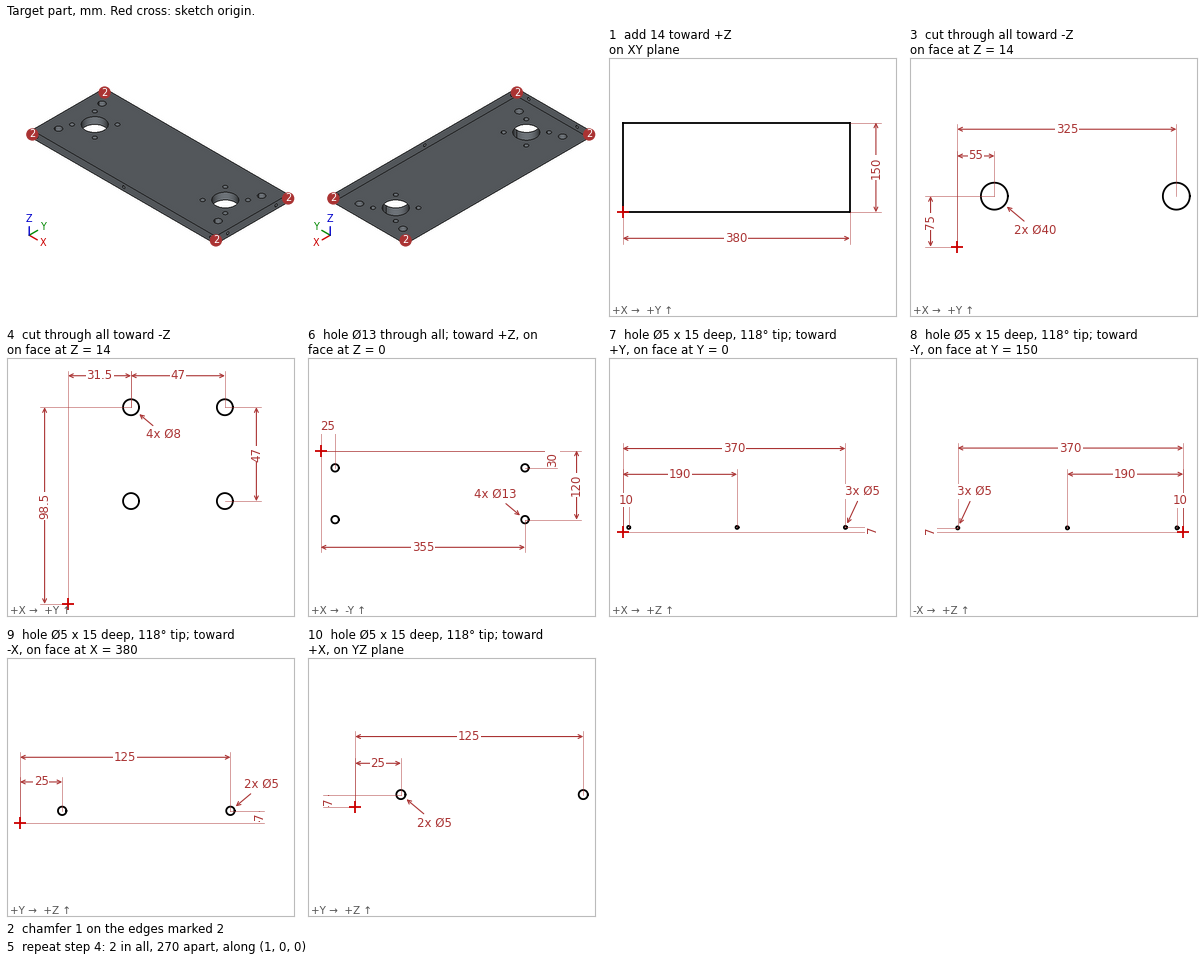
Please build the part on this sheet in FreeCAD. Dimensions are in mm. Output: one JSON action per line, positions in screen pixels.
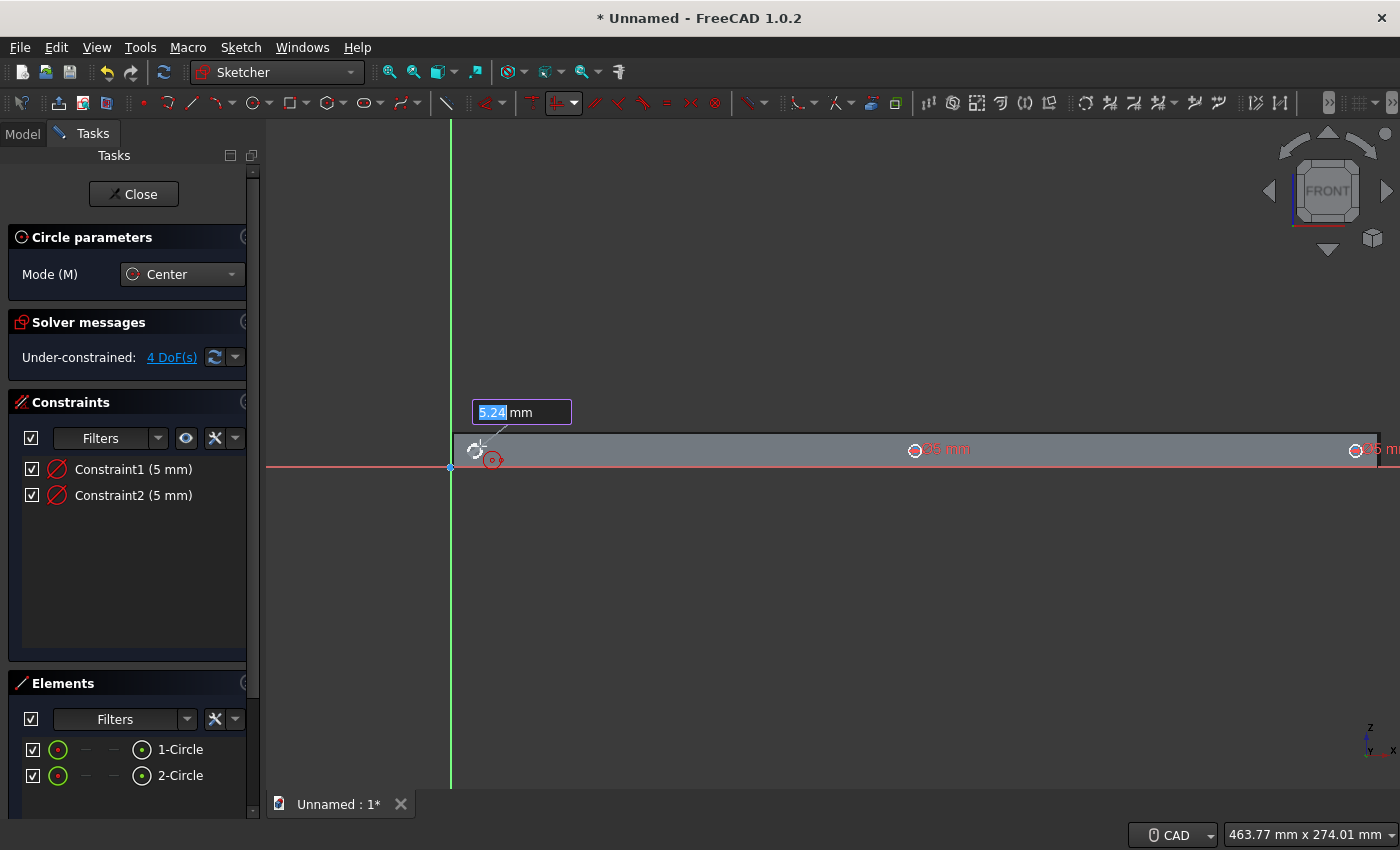
{"action": "type", "text": "5"}
{"action": "key", "text": "Return"}
{"action": "key", "text": "Escape"}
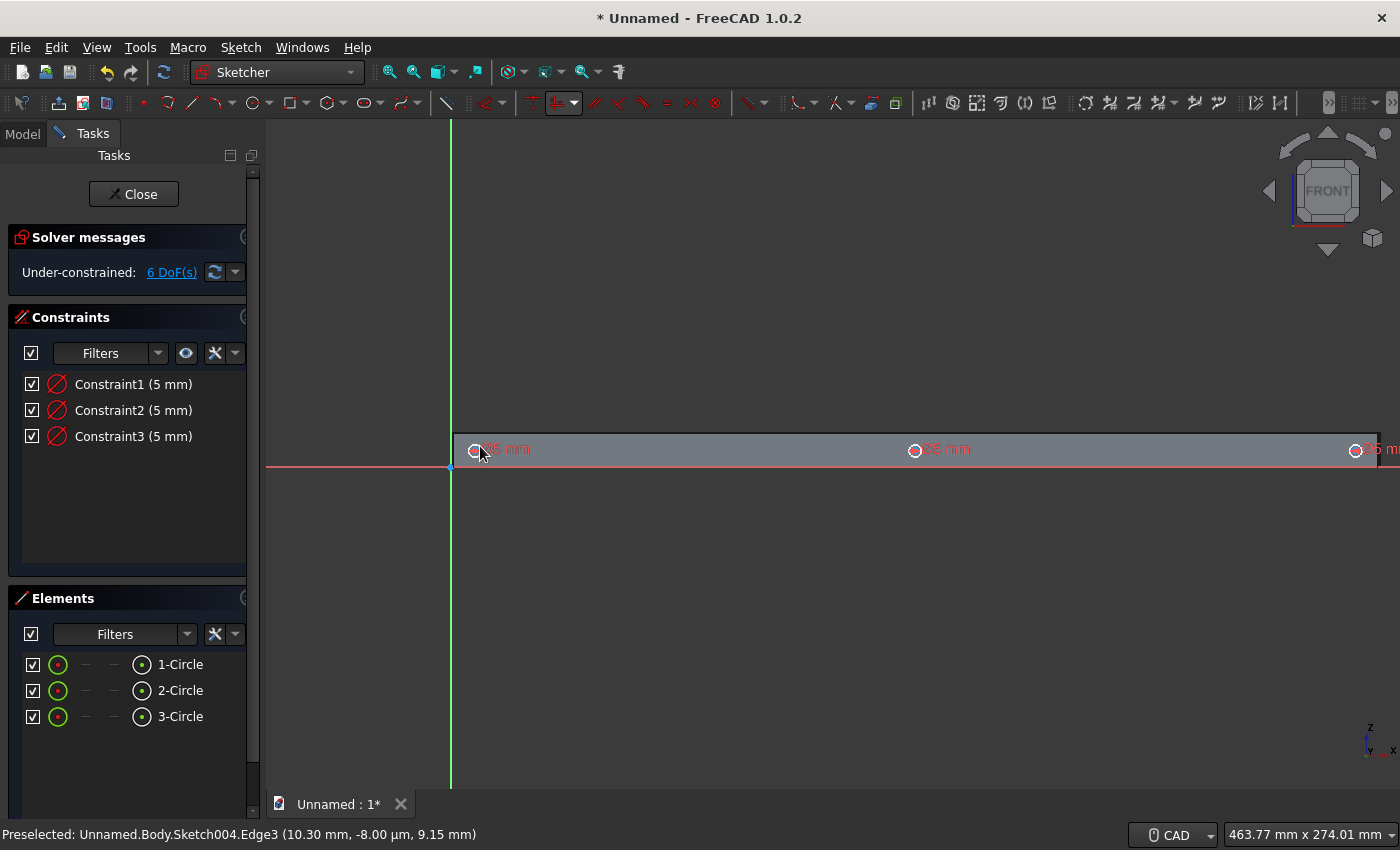
{"action": "scroll", "coordinate": [476, 450], "scroll_direction": "down", "scroll_amount": 2}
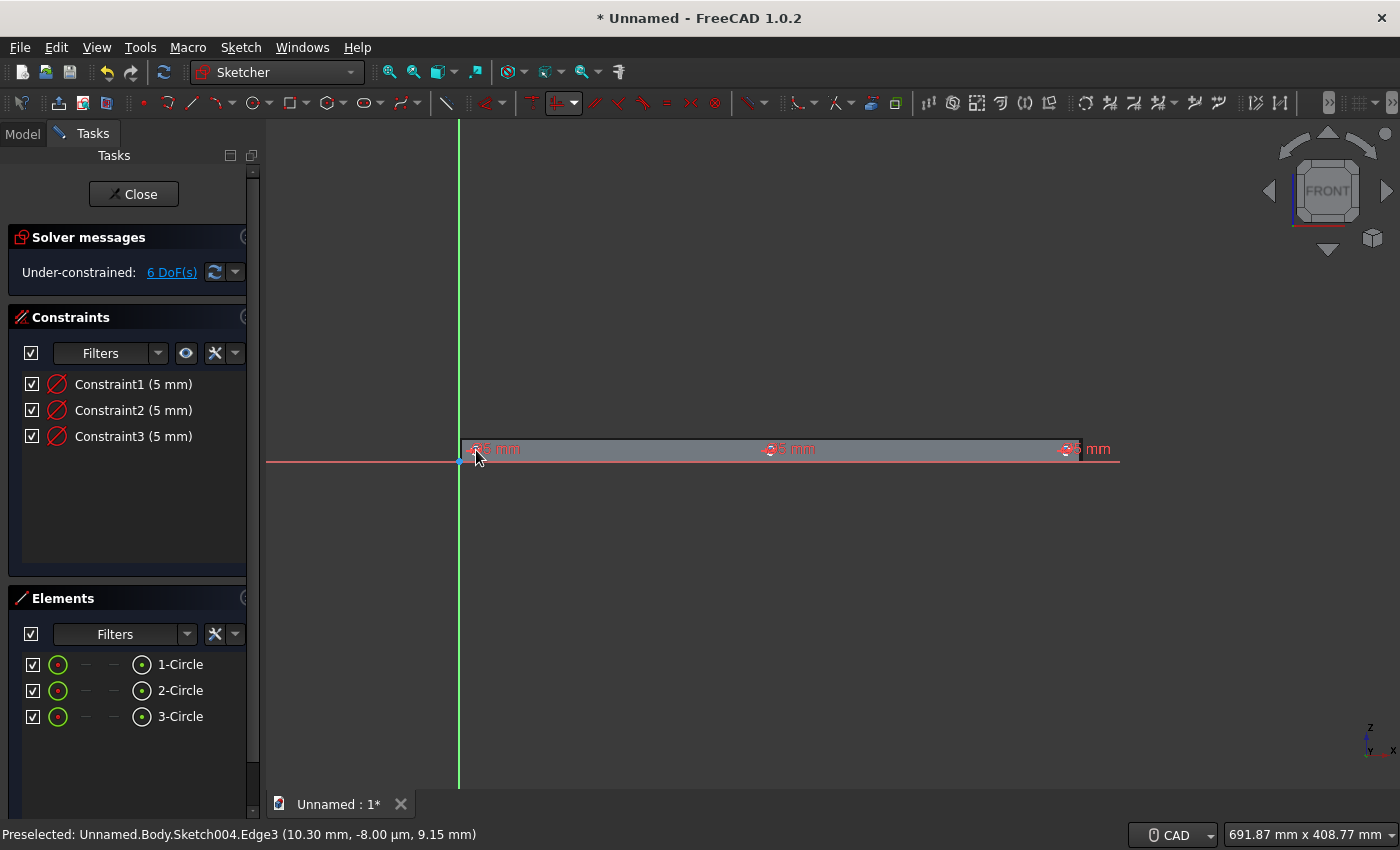
{"action": "left_click", "coordinate": [1066, 451]}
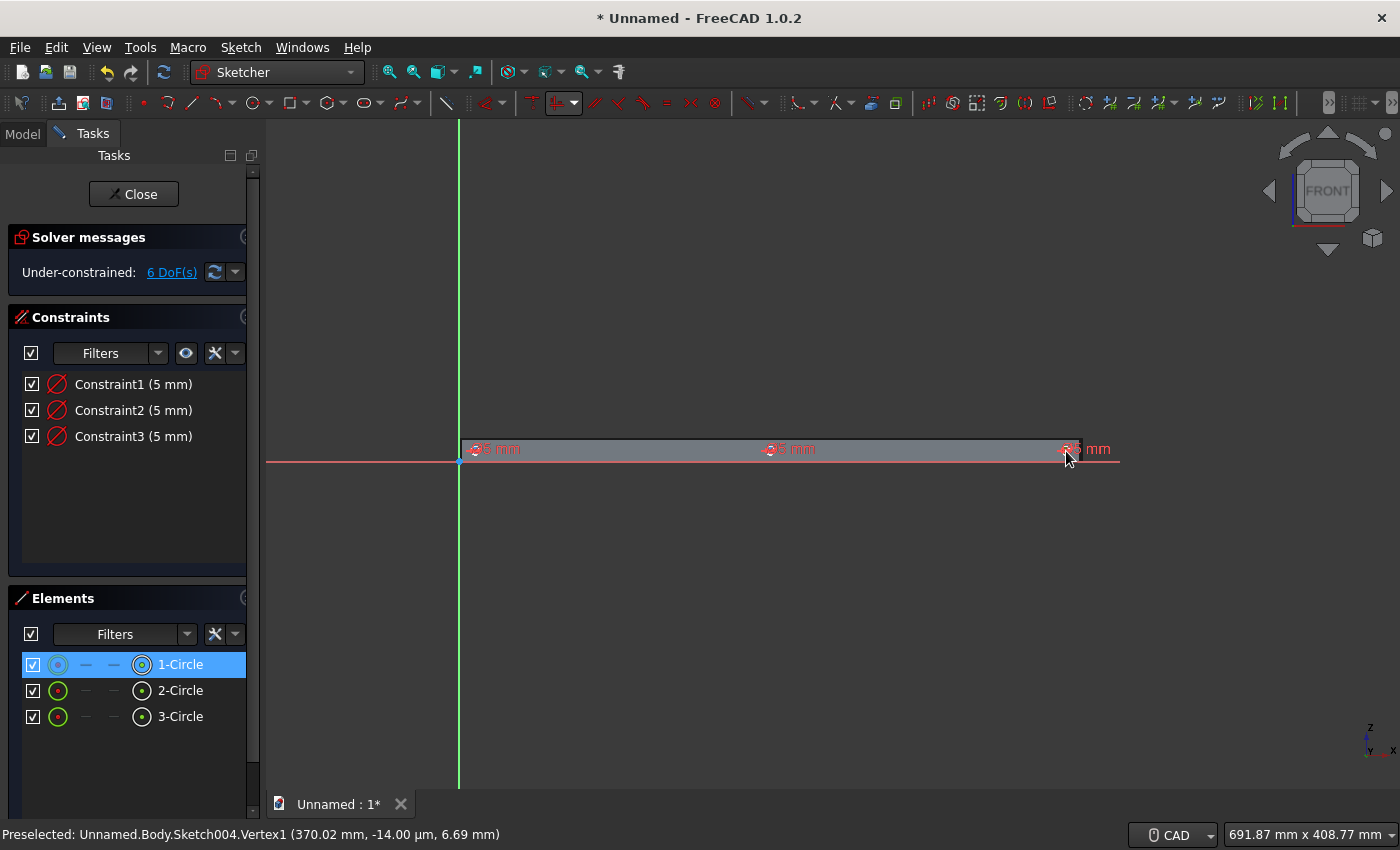
{"action": "left_click", "coordinate": [770, 451]}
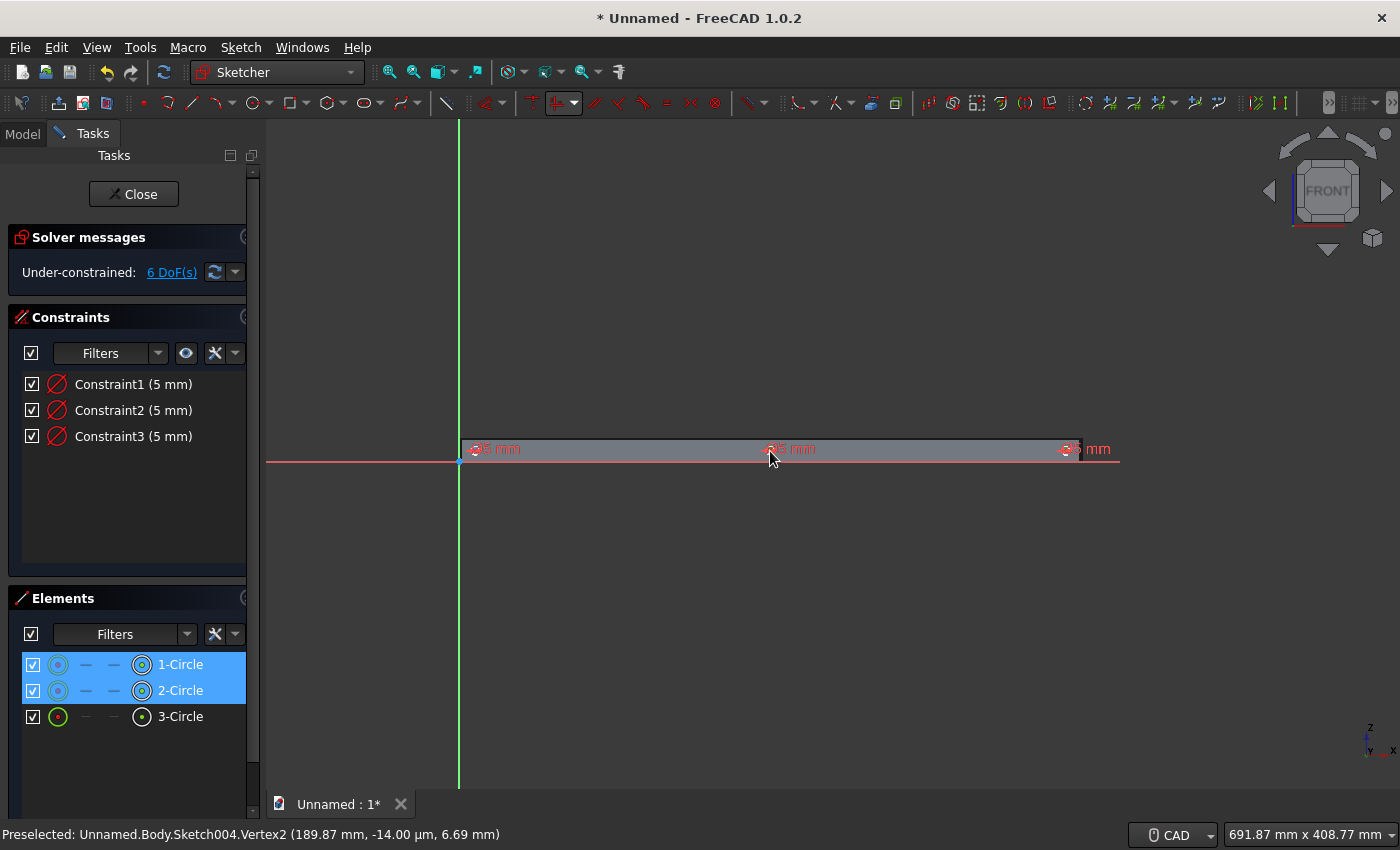
{"action": "key", "text": "h"}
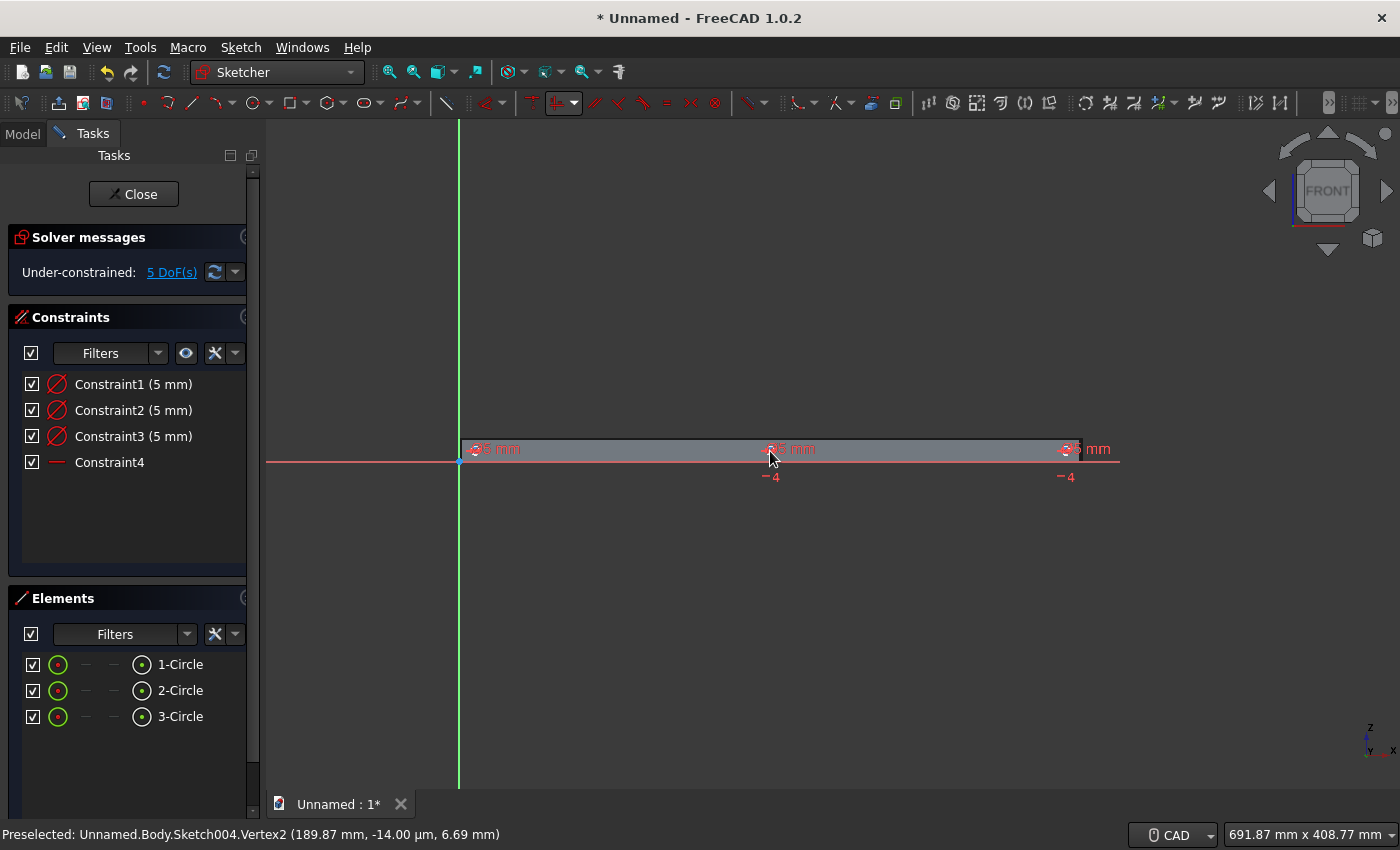
{"action": "left_click", "coordinate": [770, 451]}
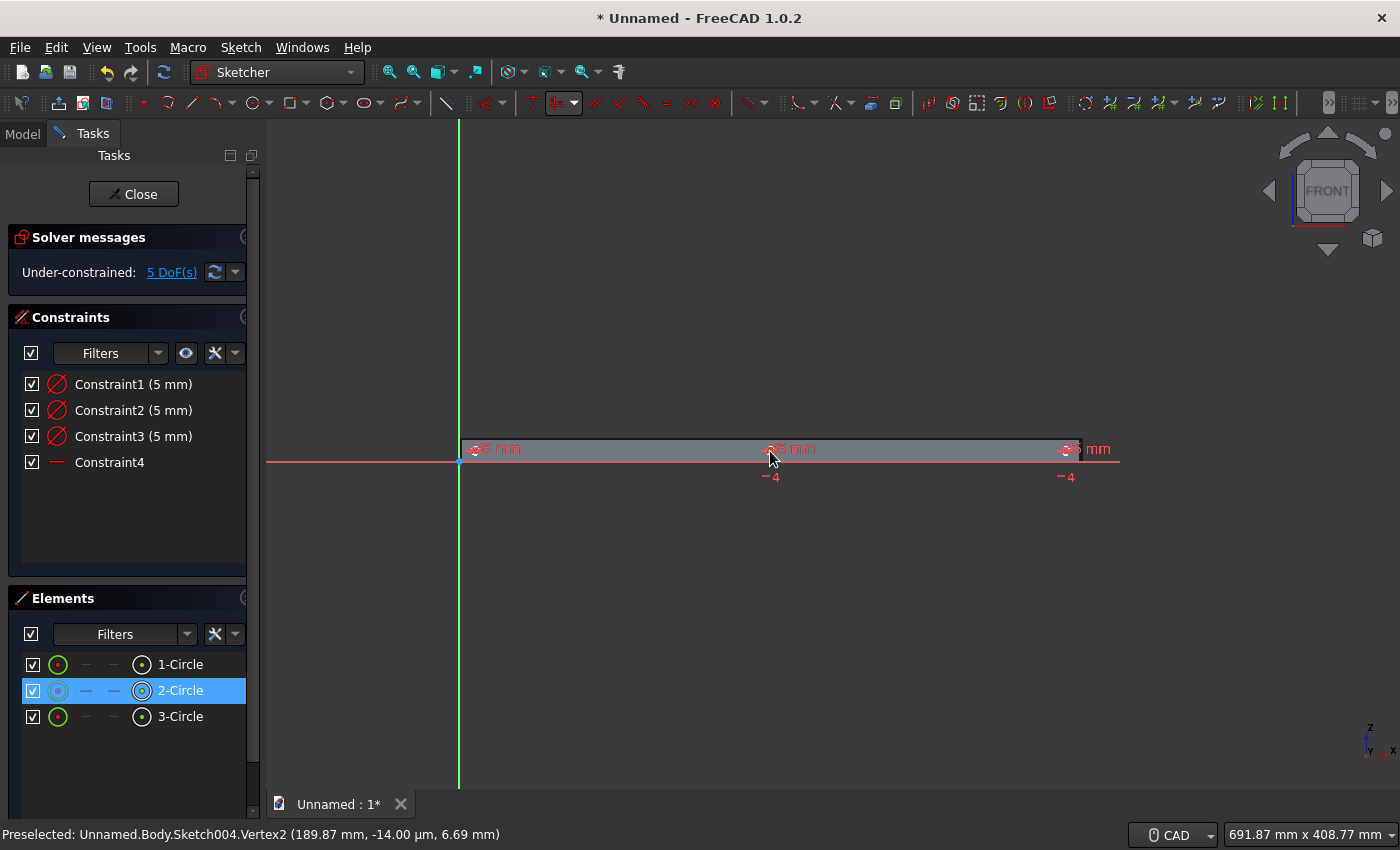
{"action": "left_click", "coordinate": [475, 451]}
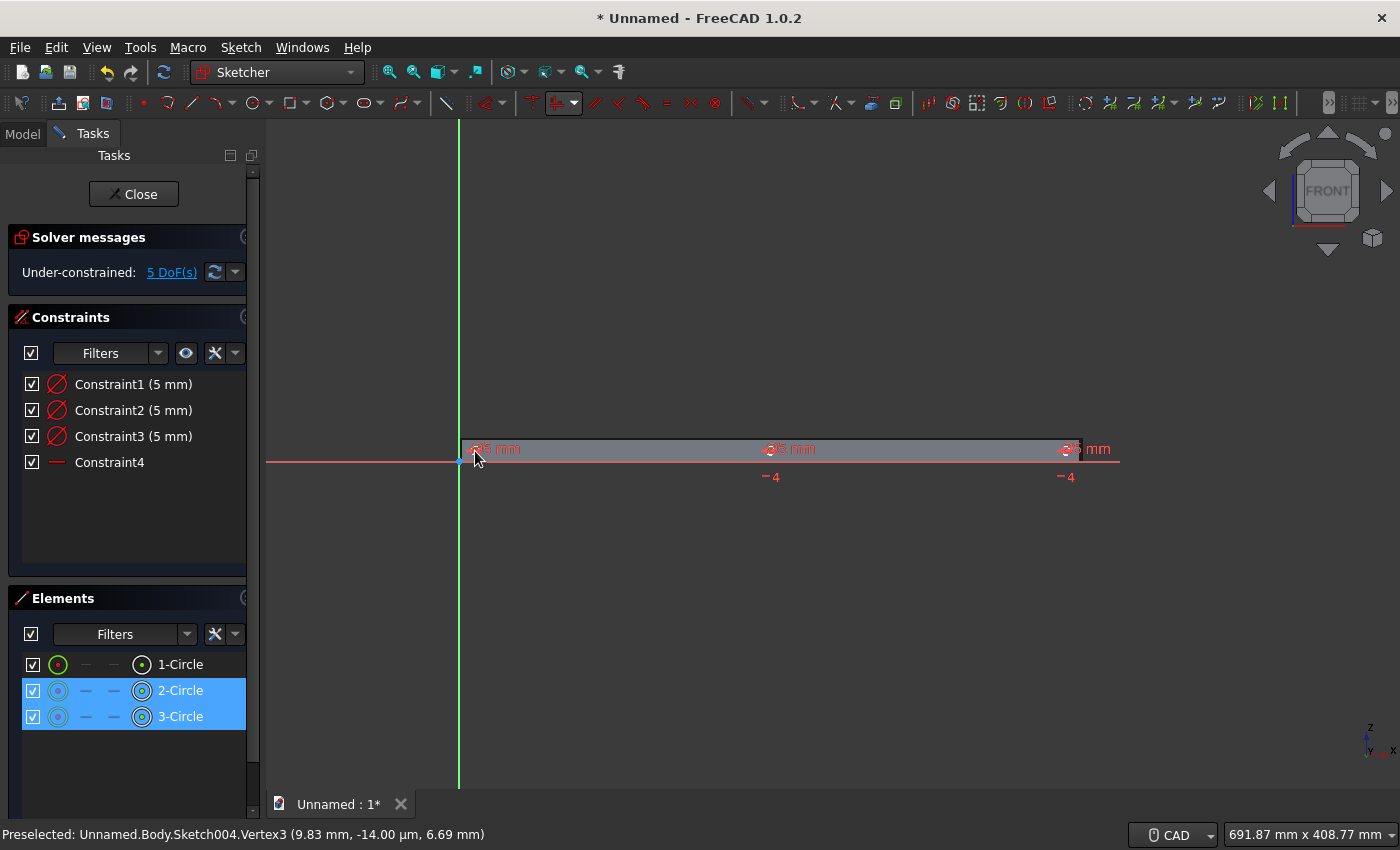
{"action": "key", "text": "h"}